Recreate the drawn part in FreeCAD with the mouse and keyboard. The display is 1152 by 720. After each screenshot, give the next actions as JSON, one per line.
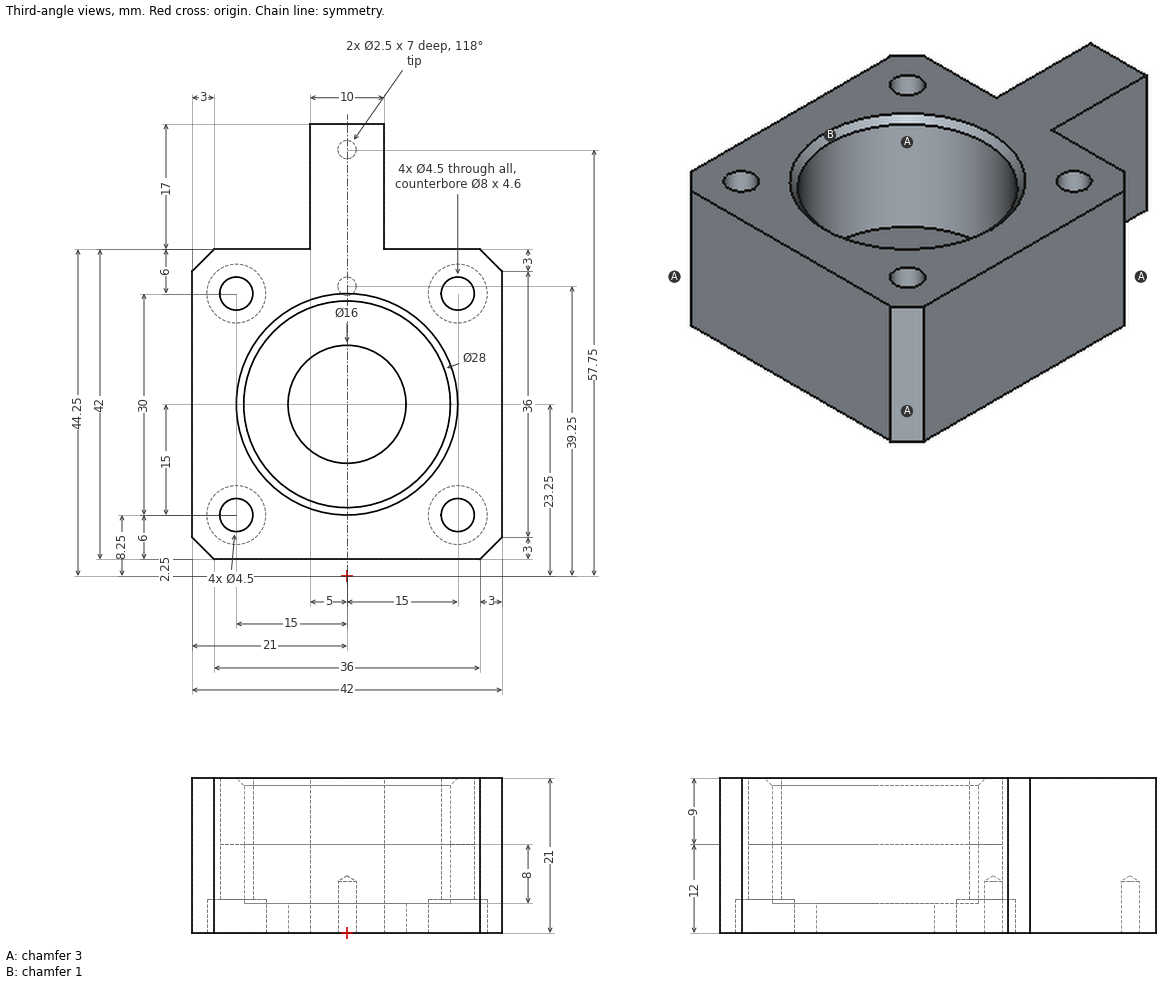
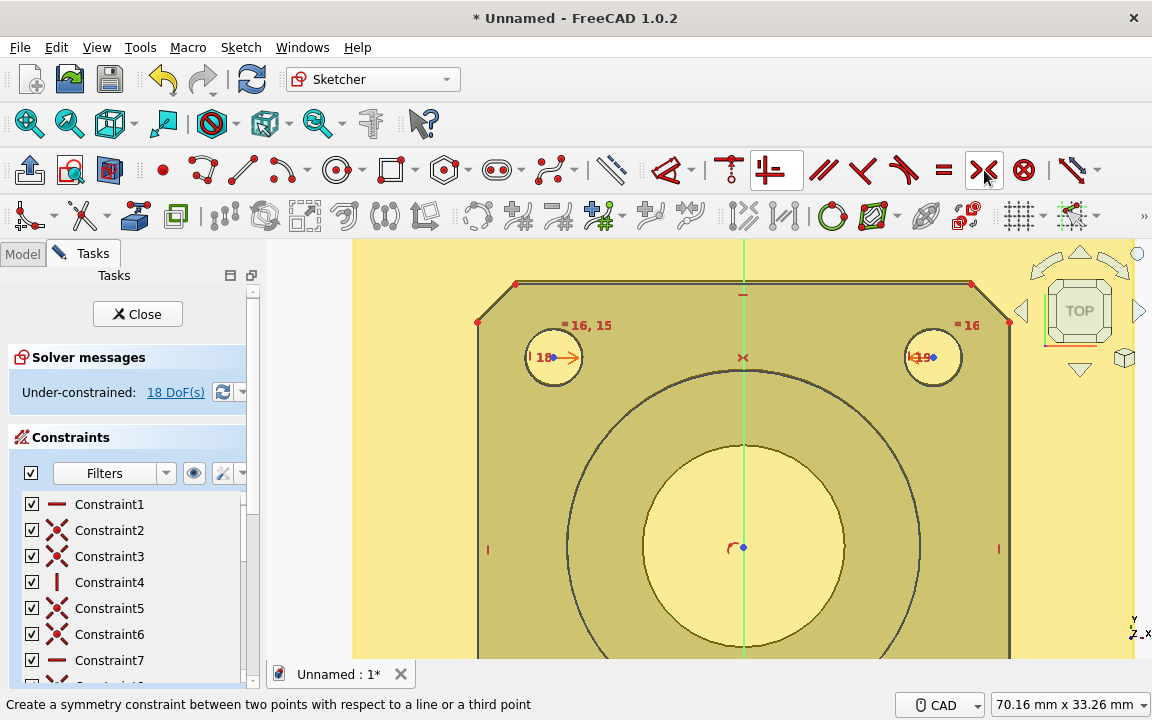
{"action": "scroll", "coordinate": [556, 358], "scroll_direction": "down", "scroll_amount": 4}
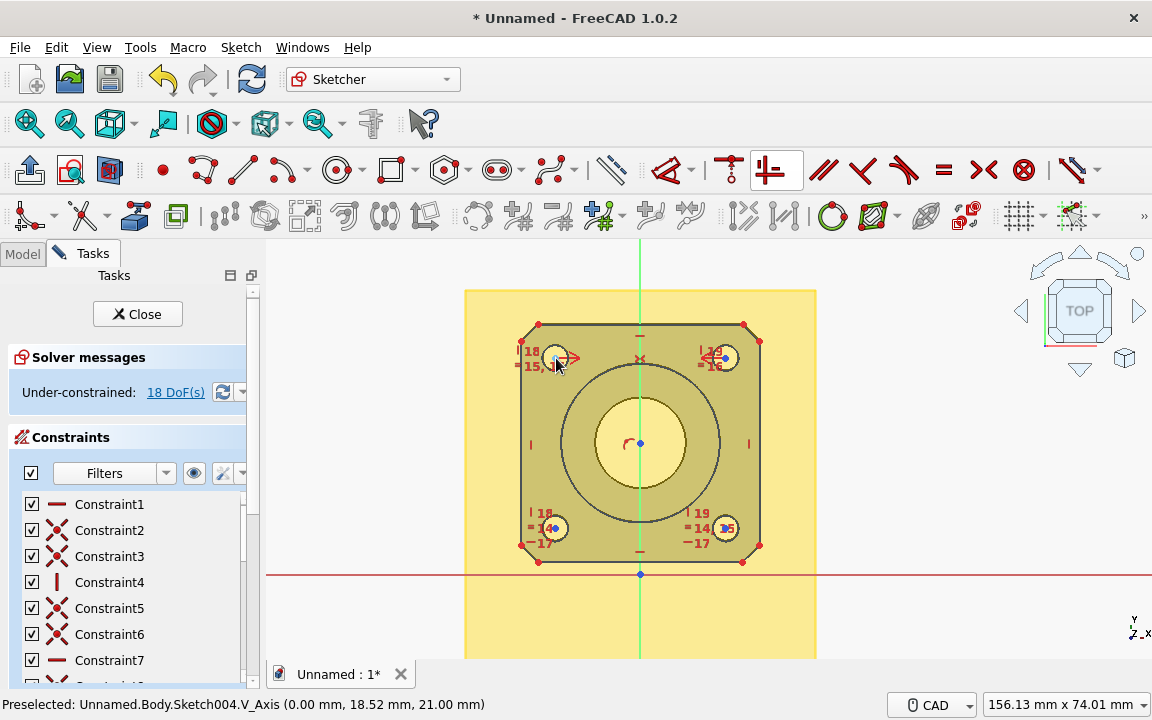
{"action": "left_click", "coordinate": [760, 342]}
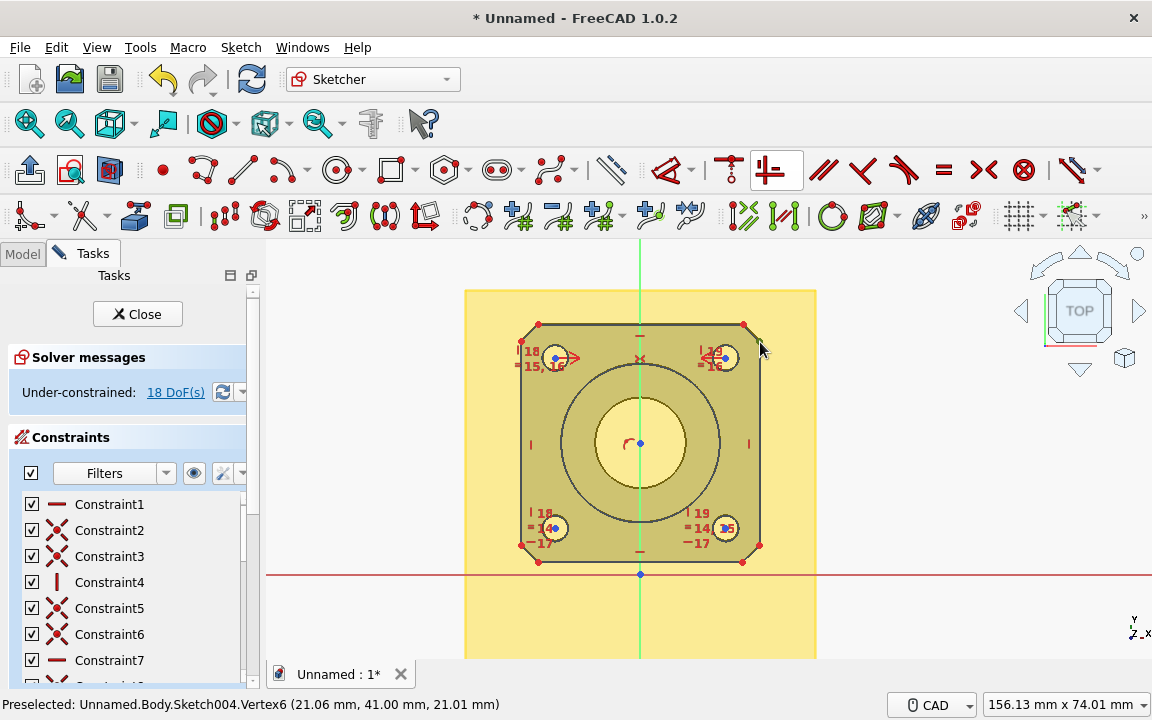
{"action": "left_click", "coordinate": [521, 342]}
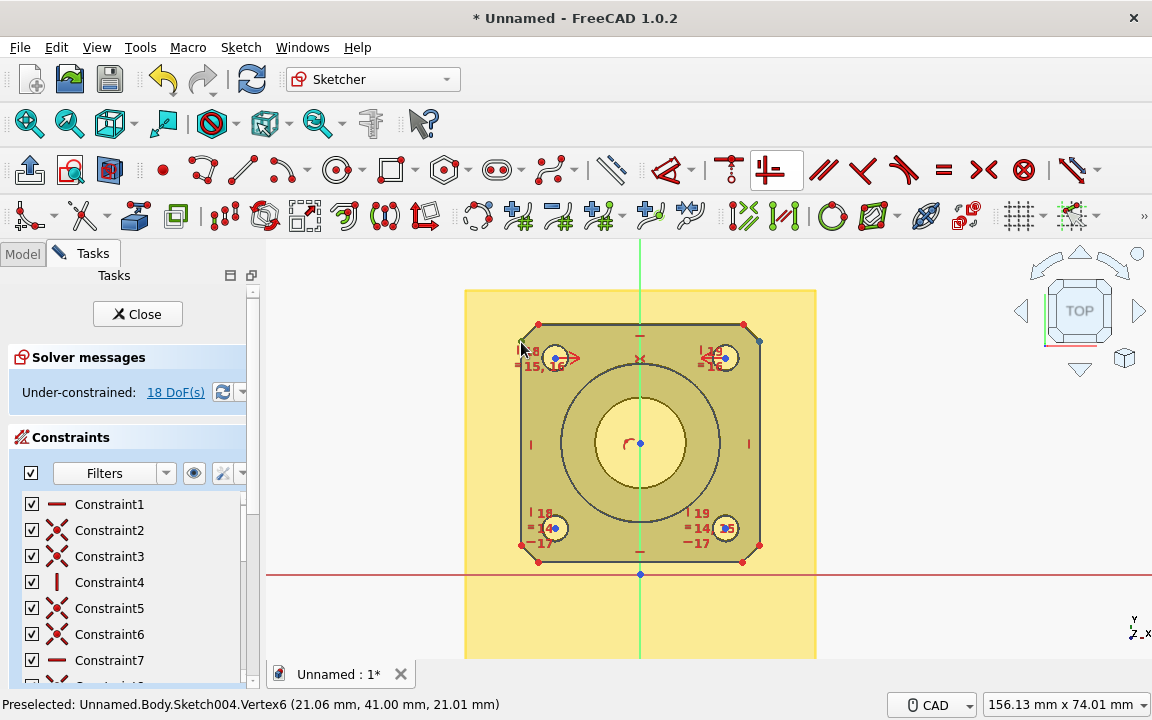
{"action": "left_click", "coordinate": [640, 605]}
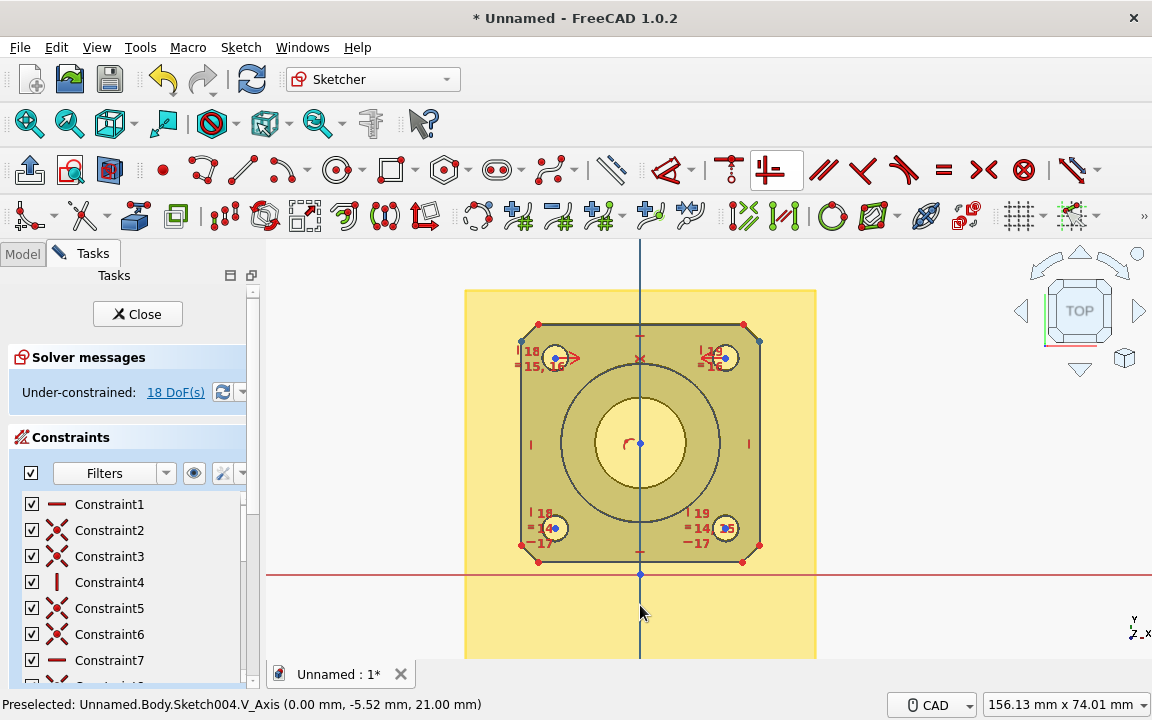
{"action": "left_click", "coordinate": [984, 170]}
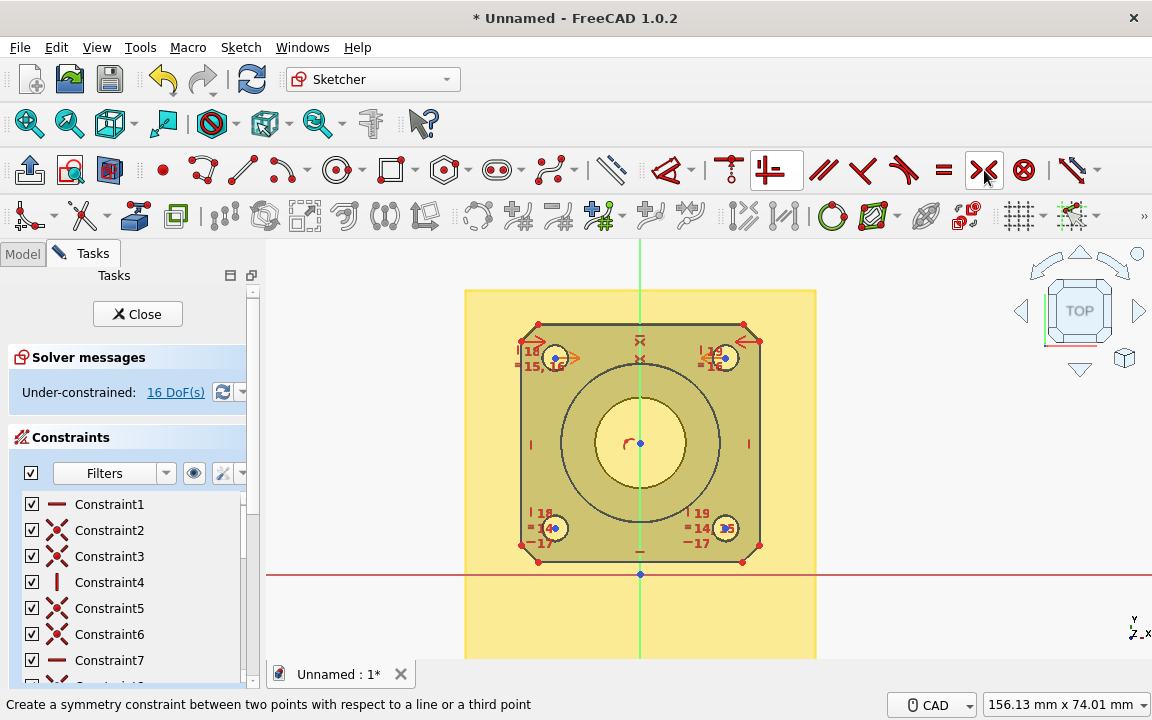
{"action": "left_click", "coordinate": [666, 170]}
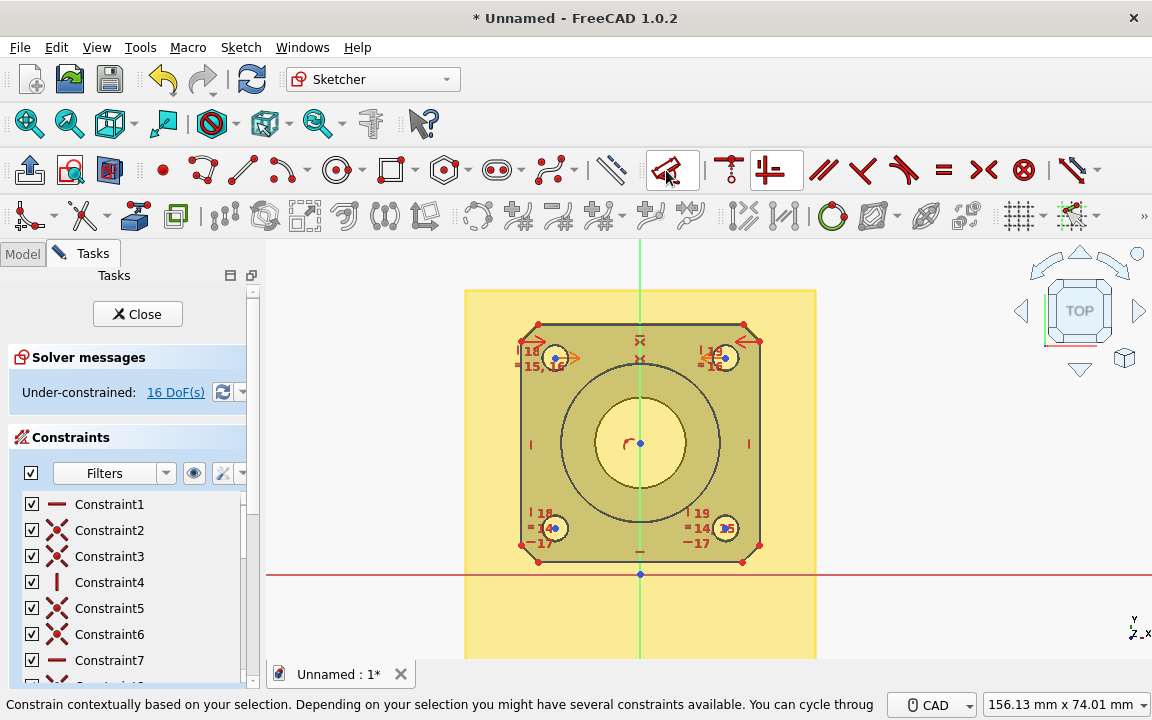
{"action": "scroll", "coordinate": [564, 520], "scroll_direction": "up", "scroll_amount": 3}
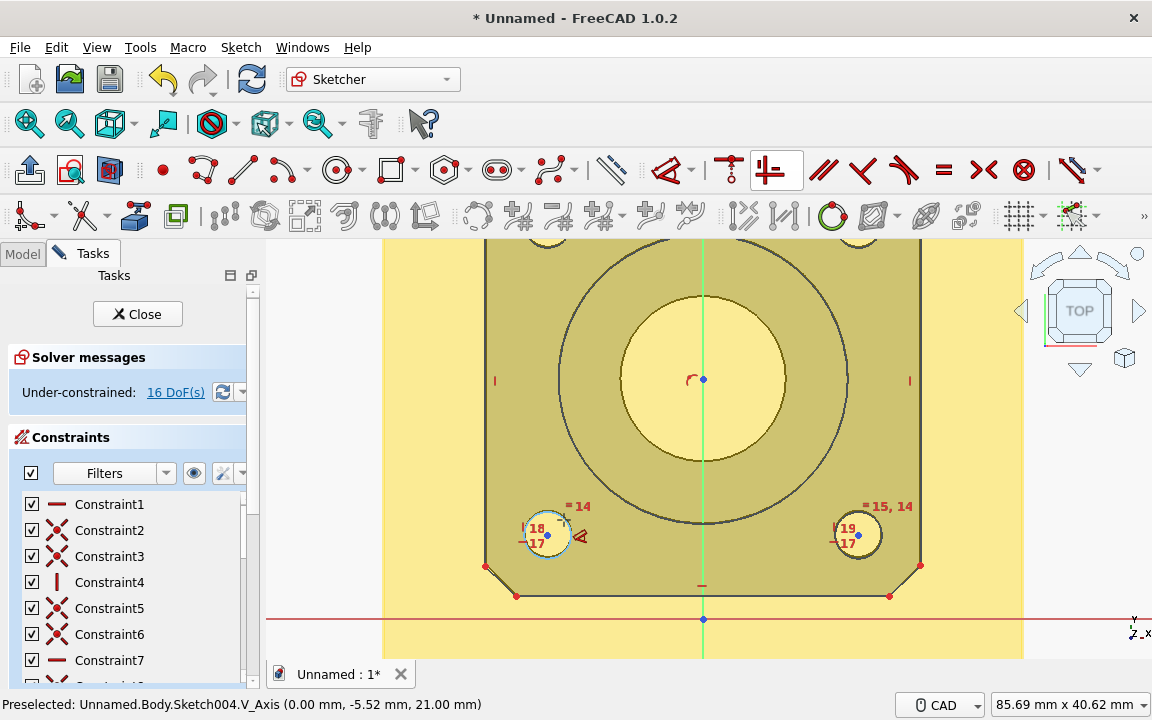
{"action": "left_click", "coordinate": [564, 519]}
{"action": "left_click", "coordinate": [587, 496]}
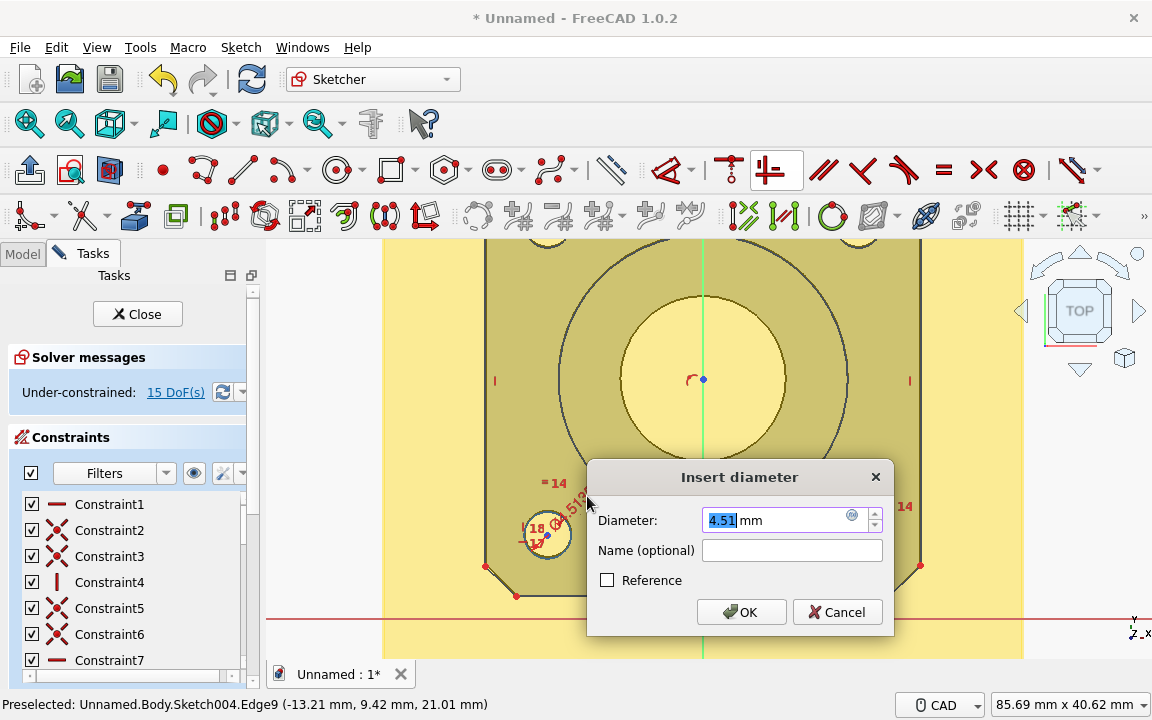
{"action": "type", "text": "4.5"}
{"action": "key", "text": "Return"}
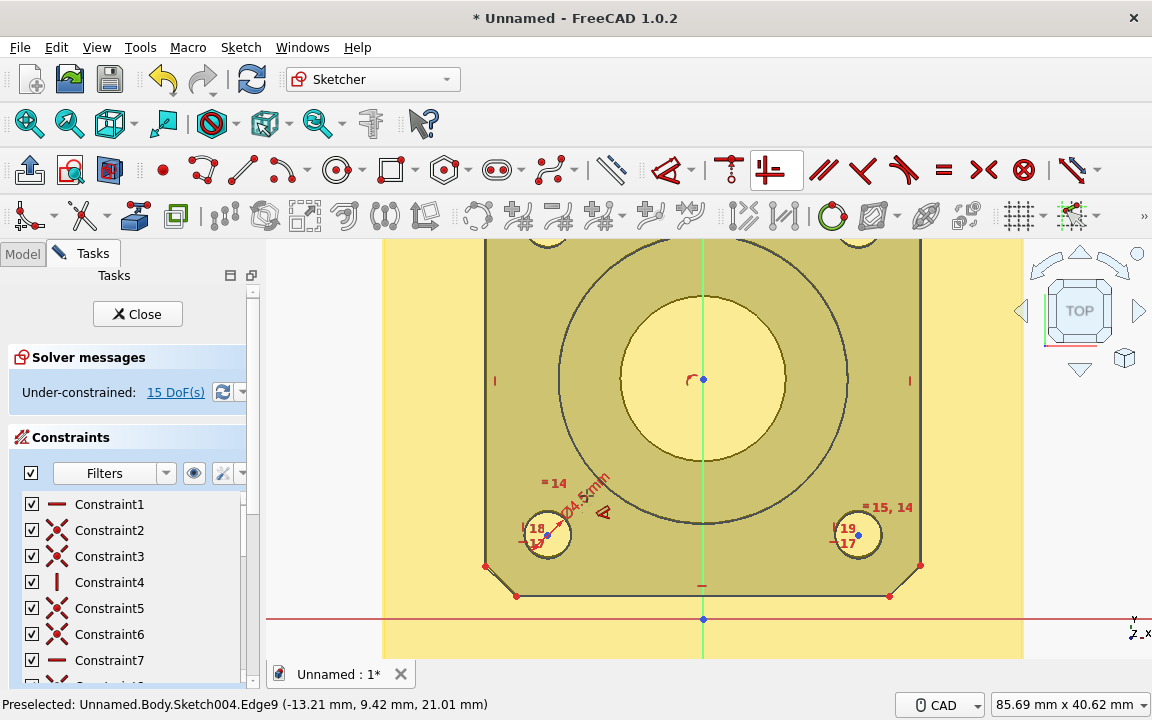
{"action": "left_click", "coordinate": [805, 277]}
{"action": "left_click", "coordinate": [872, 329]}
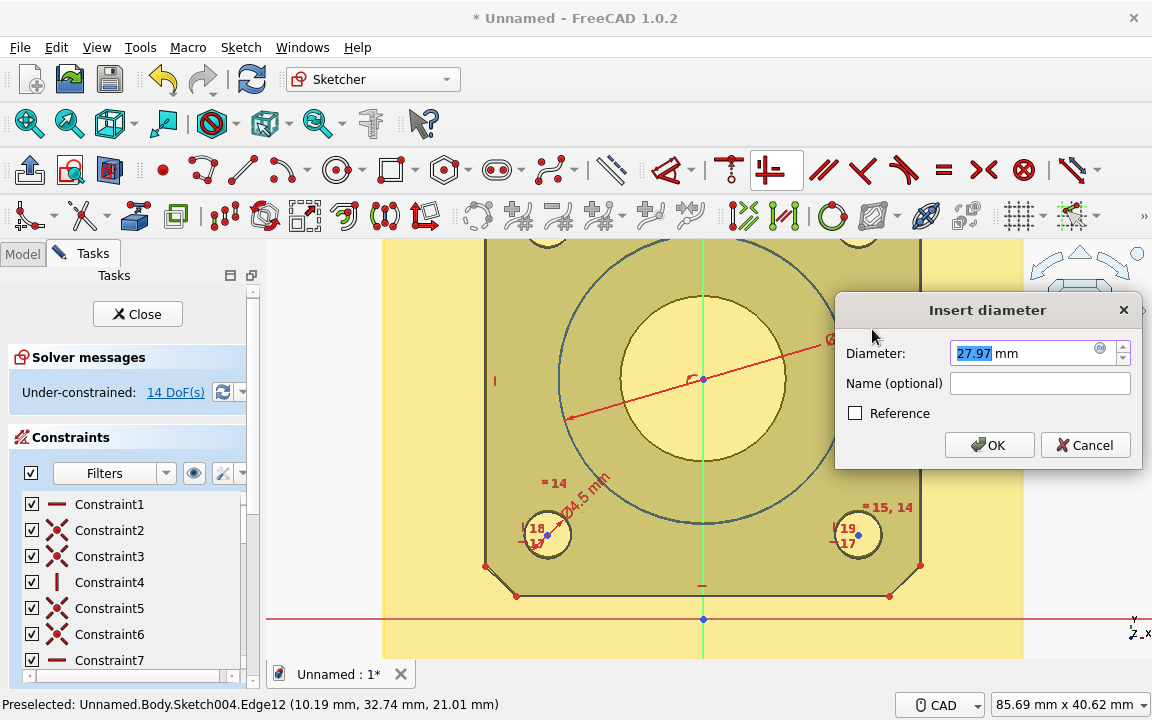
{"action": "type", "text": "28"}
{"action": "key", "text": "Return"}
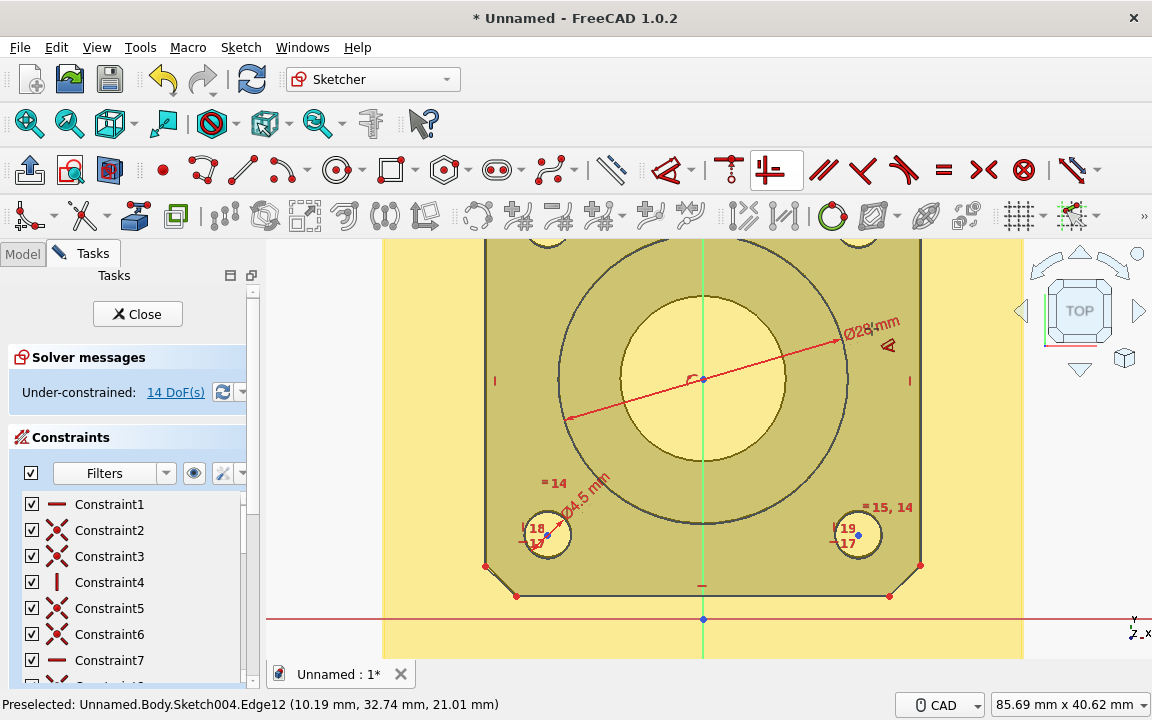
{"action": "left_click", "coordinate": [628, 596]}
{"action": "left_click", "coordinate": [617, 562]}